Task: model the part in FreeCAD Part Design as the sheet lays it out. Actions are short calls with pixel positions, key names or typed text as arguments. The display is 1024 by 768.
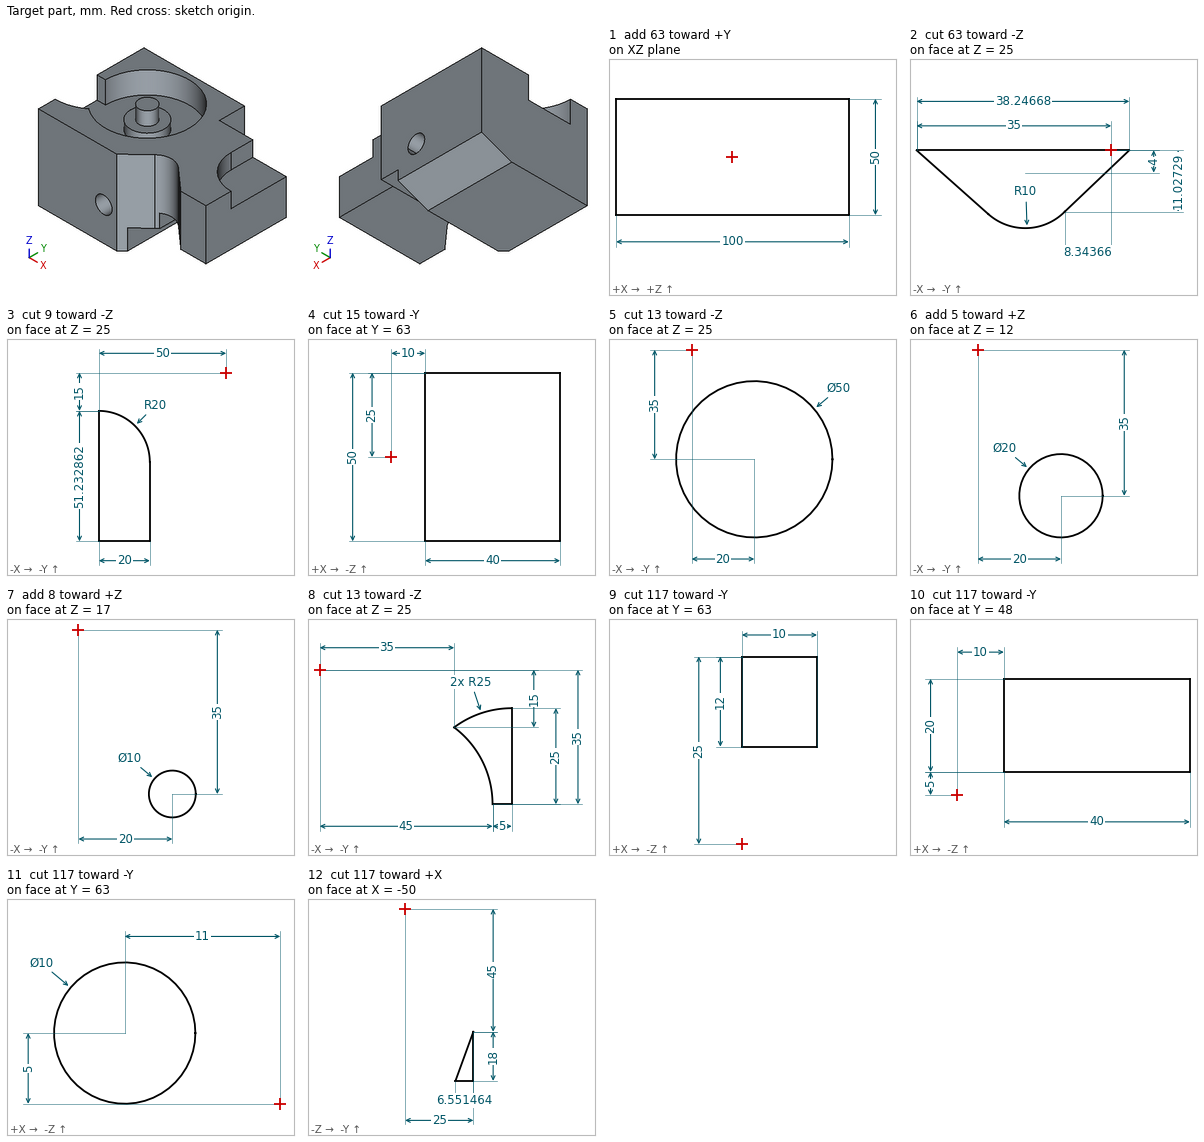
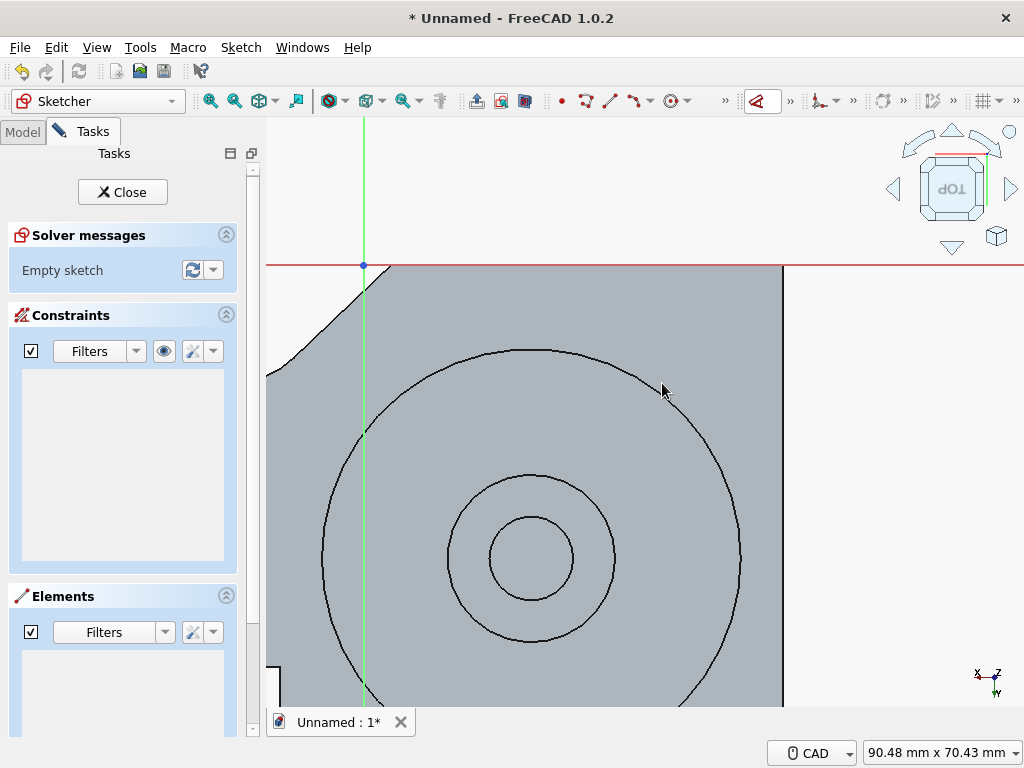
click(586, 102)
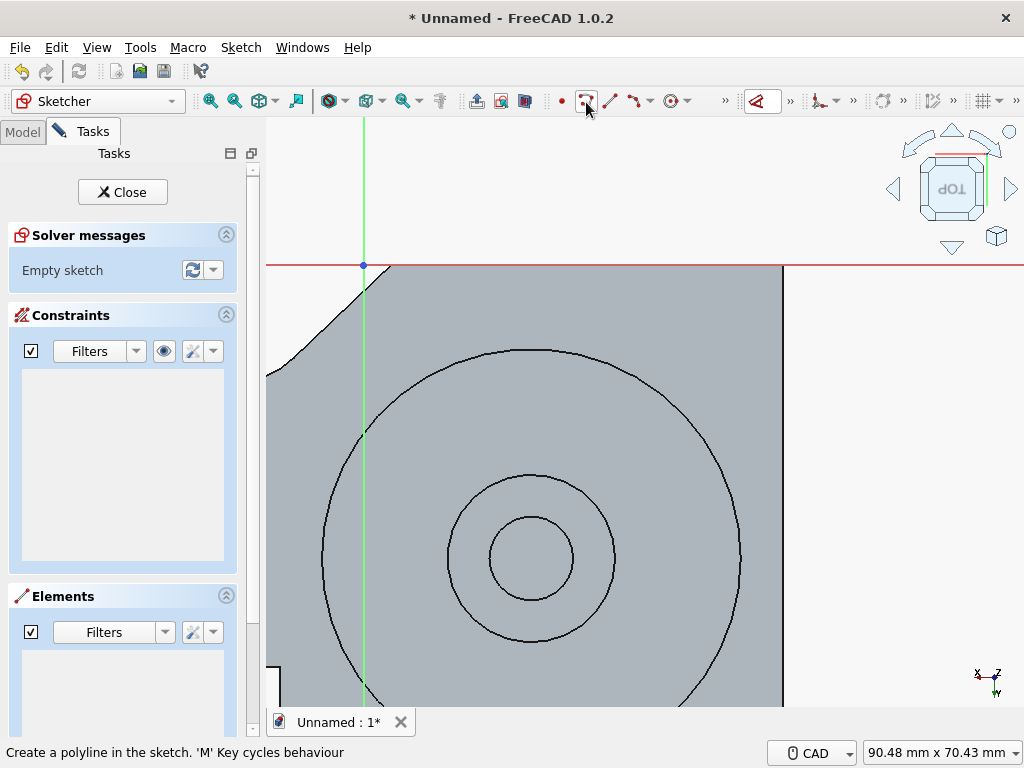
click(741, 559)
click(783, 559)
click(783, 349)
right_click(783, 349)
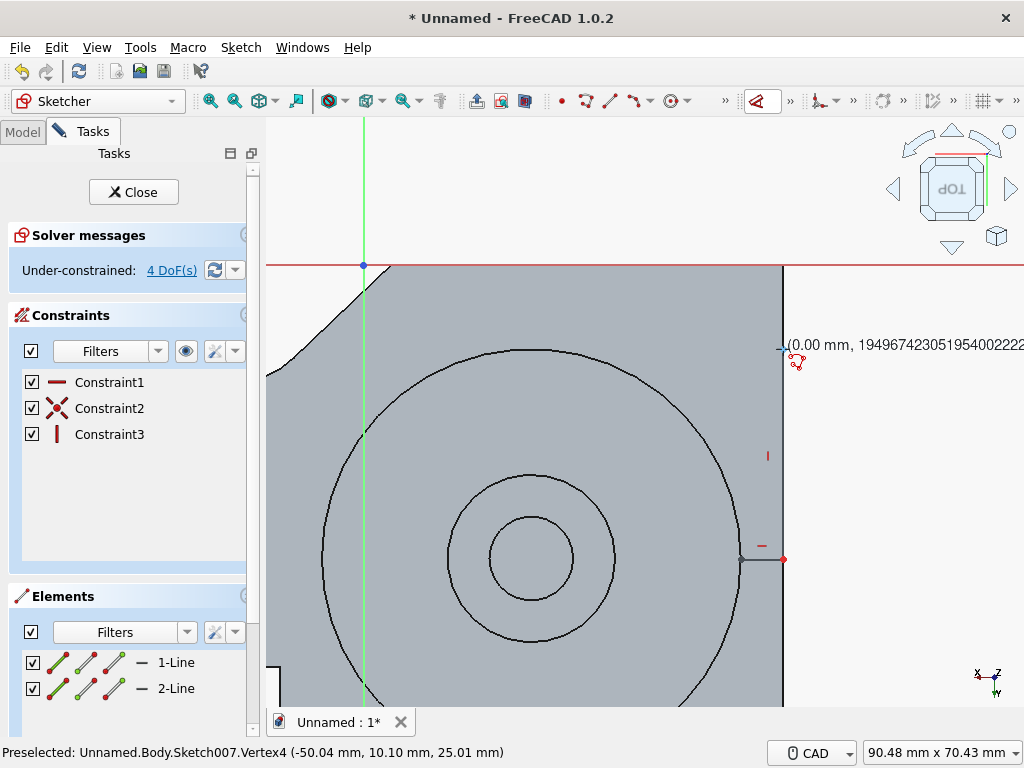
click(634, 102)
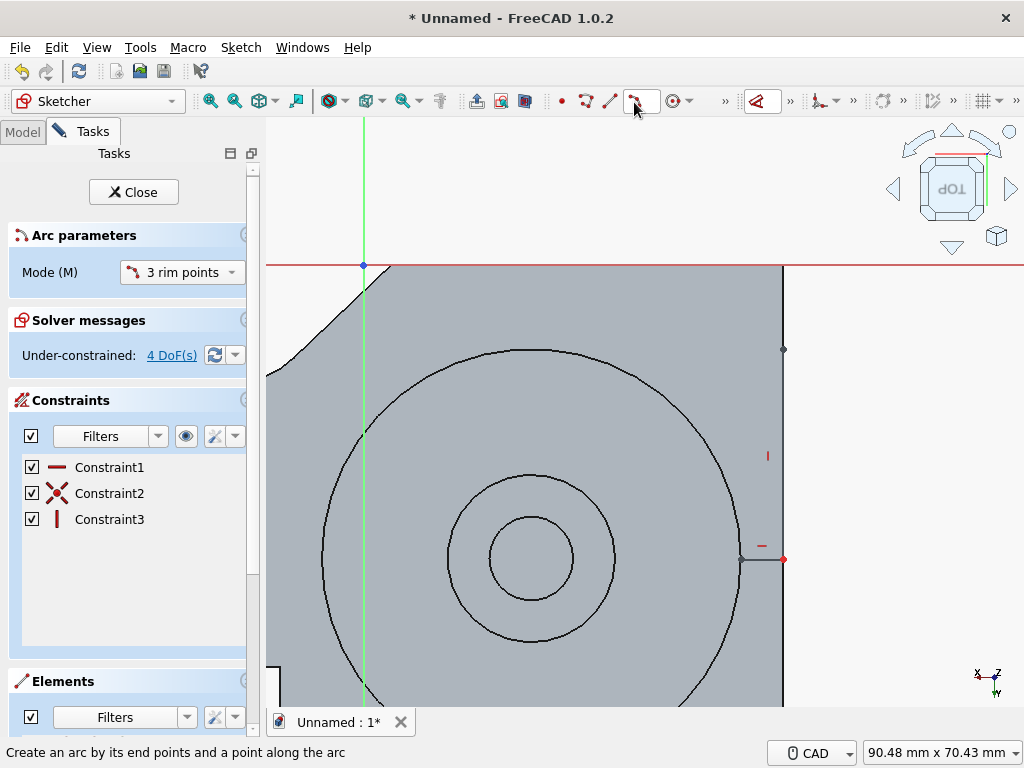
click(783, 350)
click(657, 391)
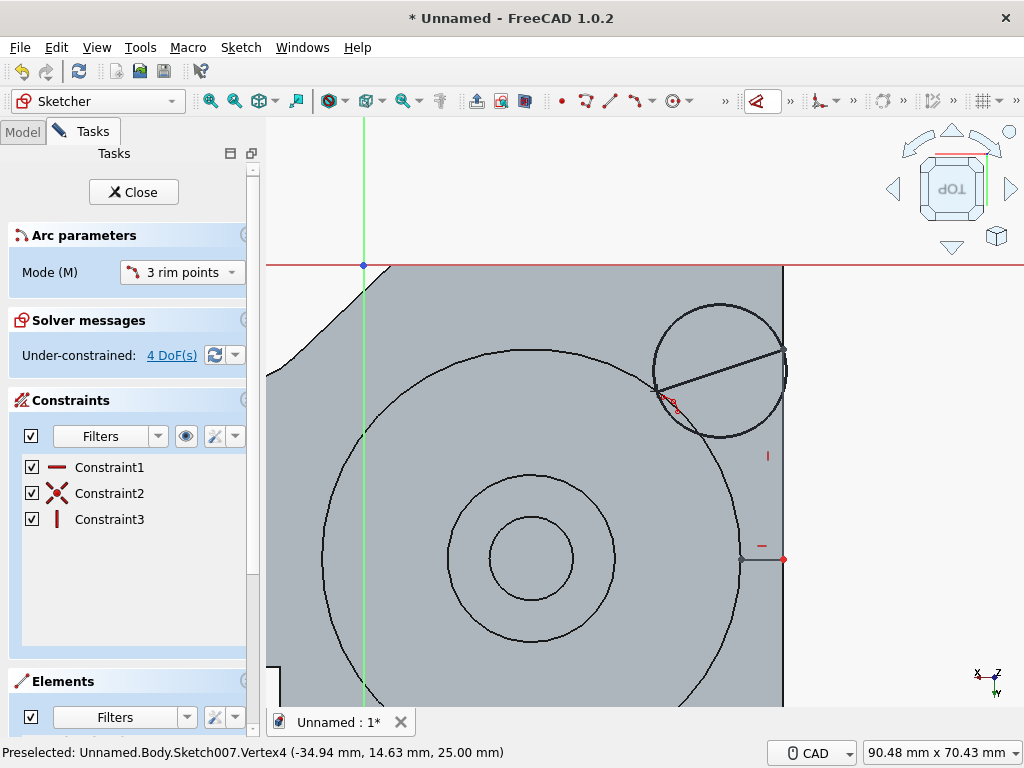
scroll(716, 360, up, 2)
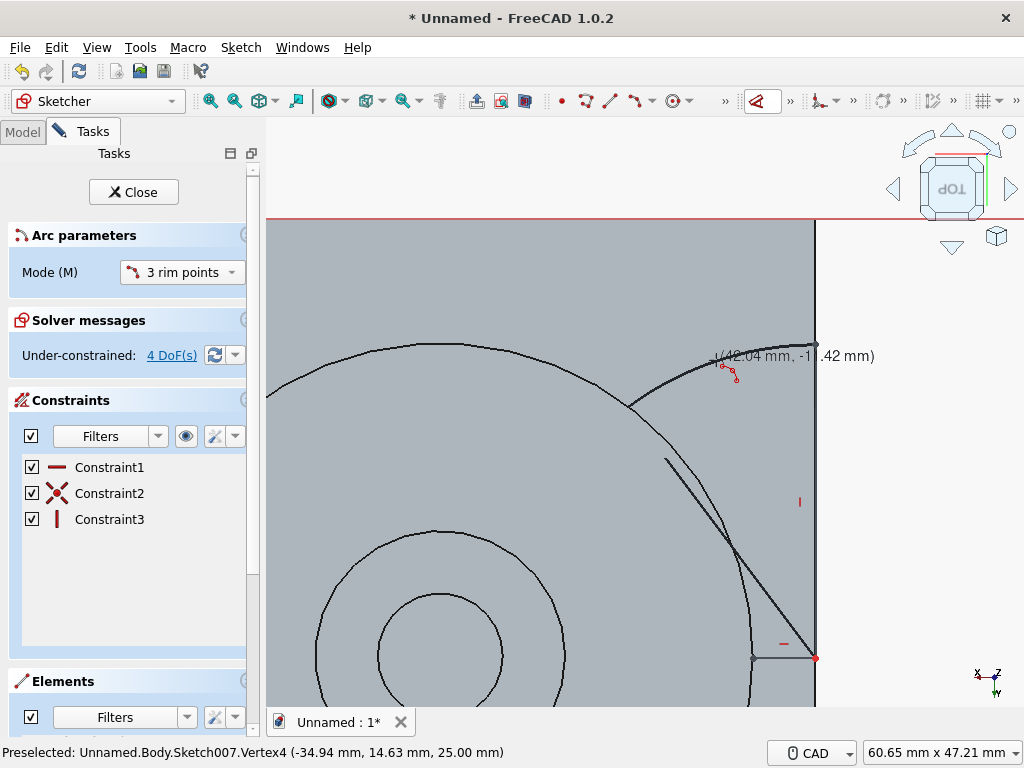
click(716, 360)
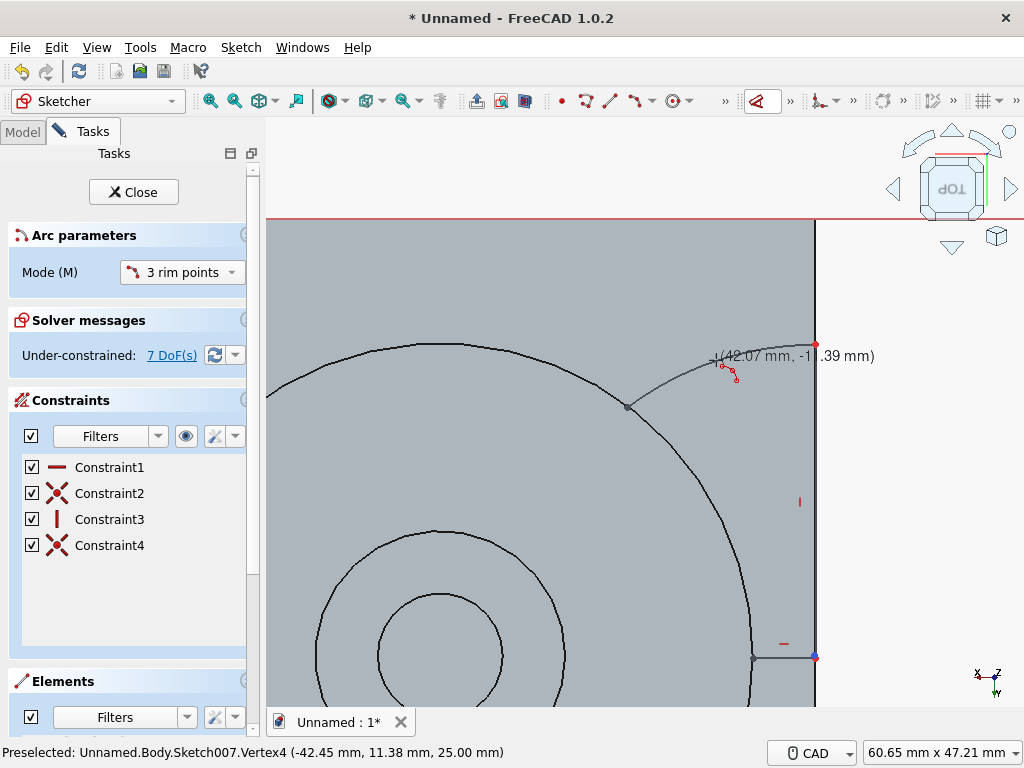
click(628, 408)
click(753, 658)
click(720, 516)
key(Escape)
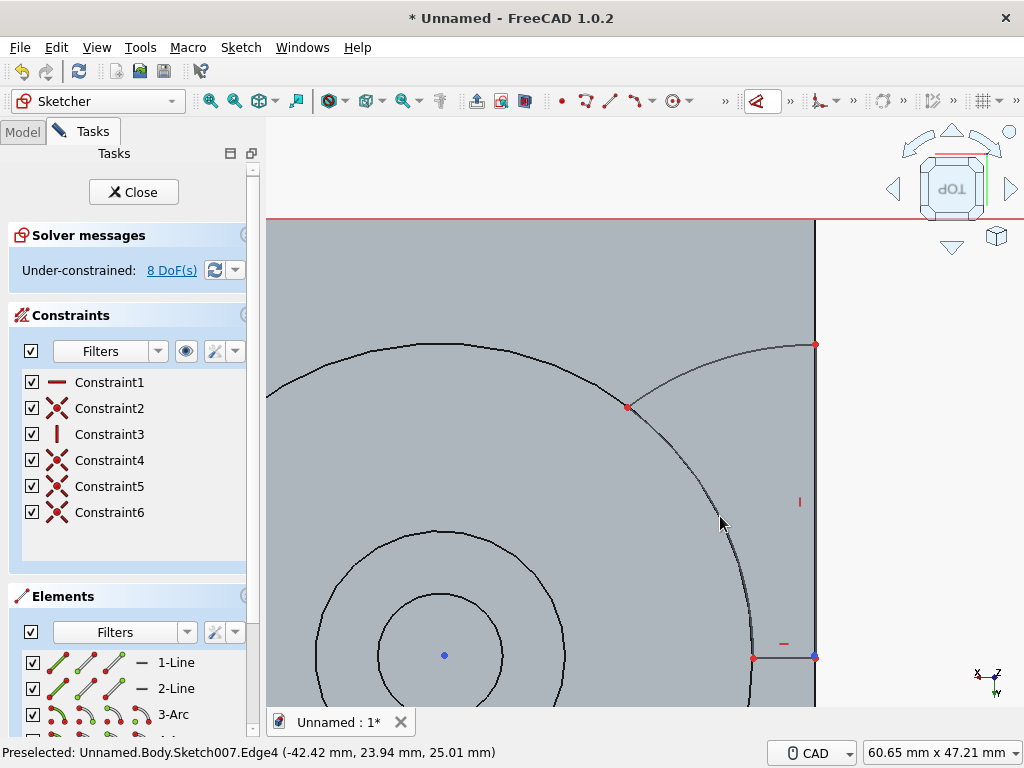
click(756, 351)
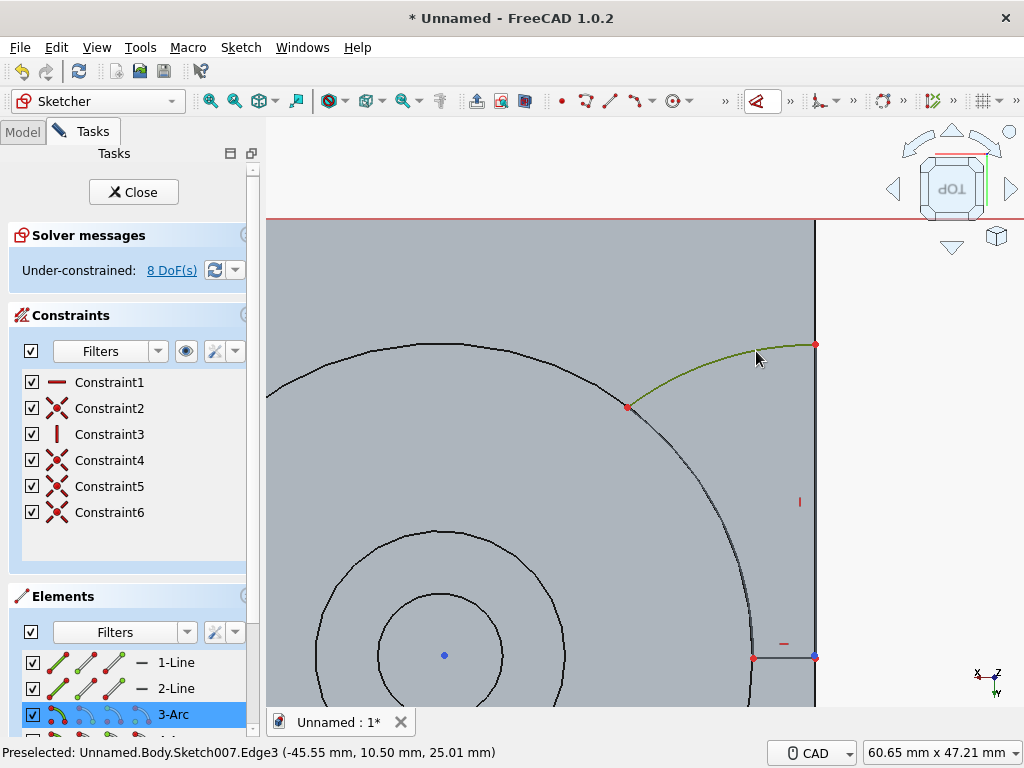
click(741, 572)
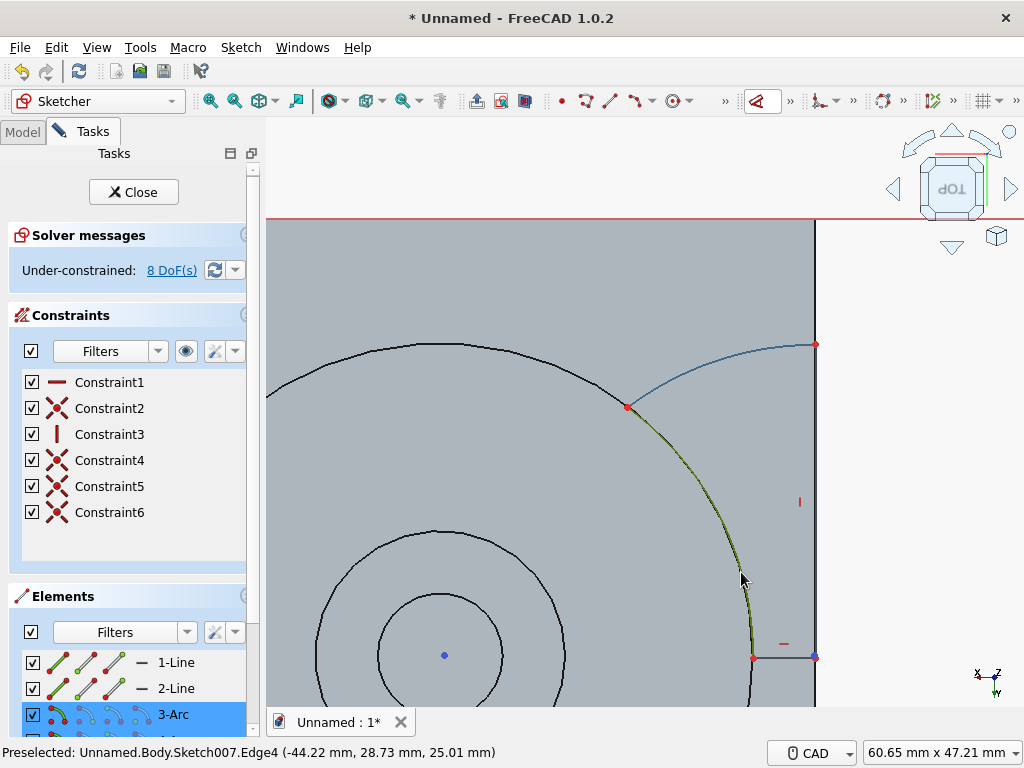
key(e)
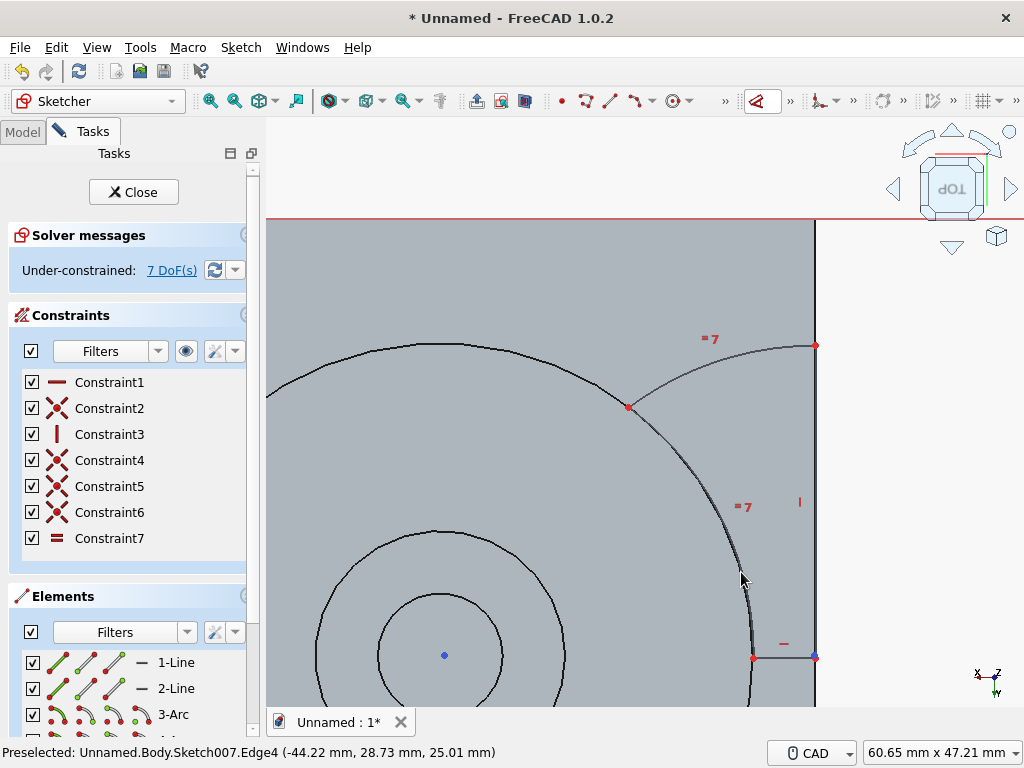
click(756, 351)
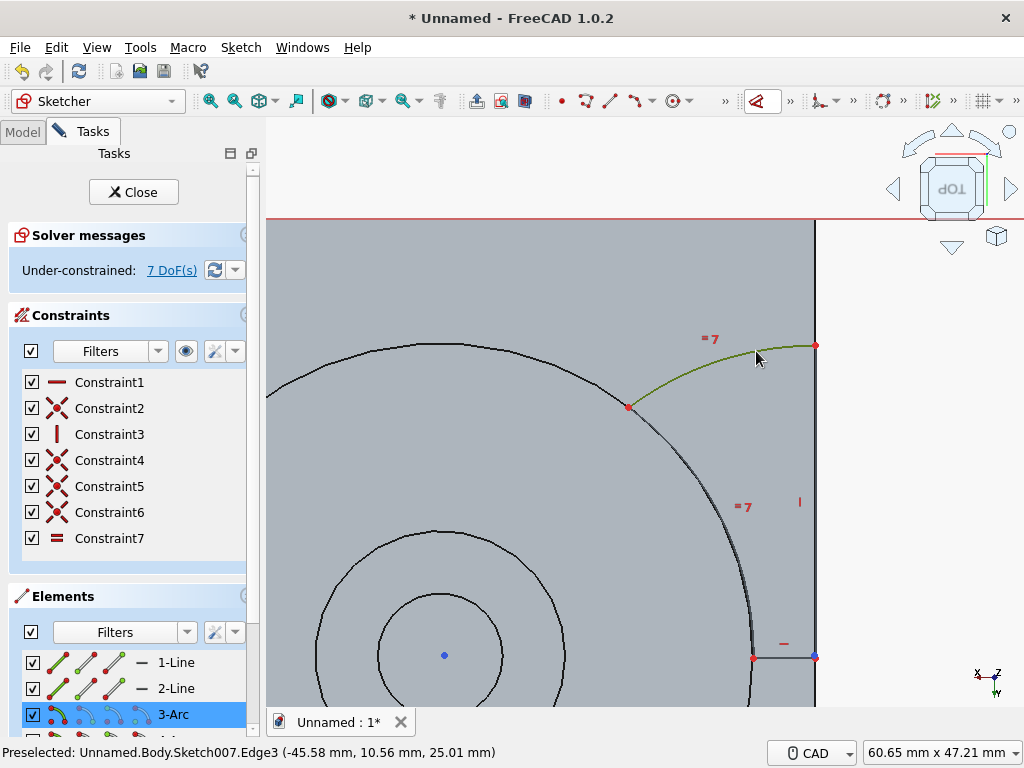
click(776, 102)